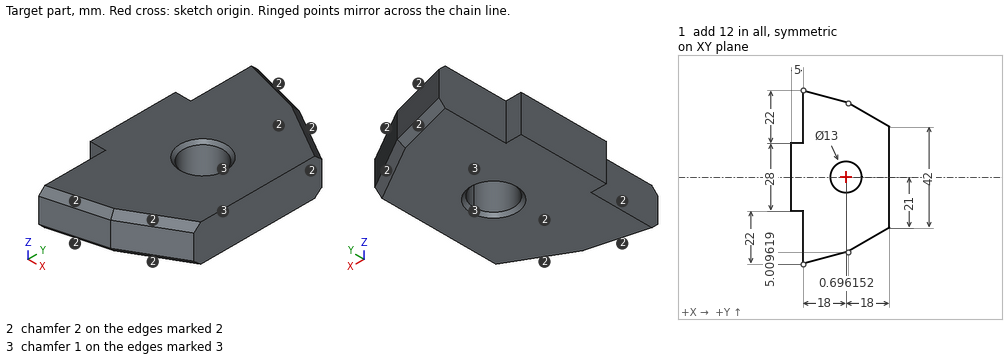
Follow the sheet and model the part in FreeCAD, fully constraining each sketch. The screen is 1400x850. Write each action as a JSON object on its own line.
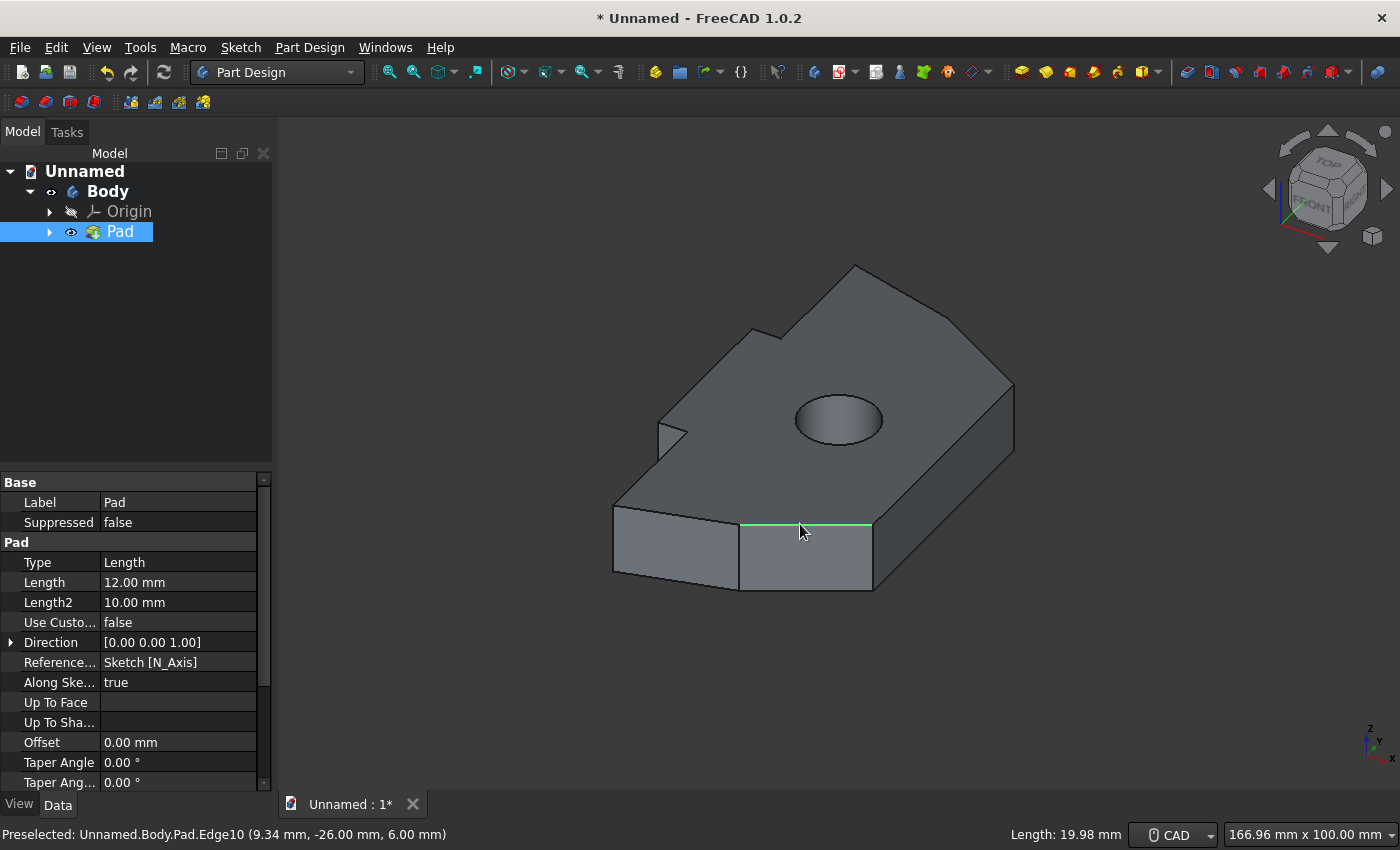
{"action": "left_click", "coordinate": [676, 514], "text": "ctrl"}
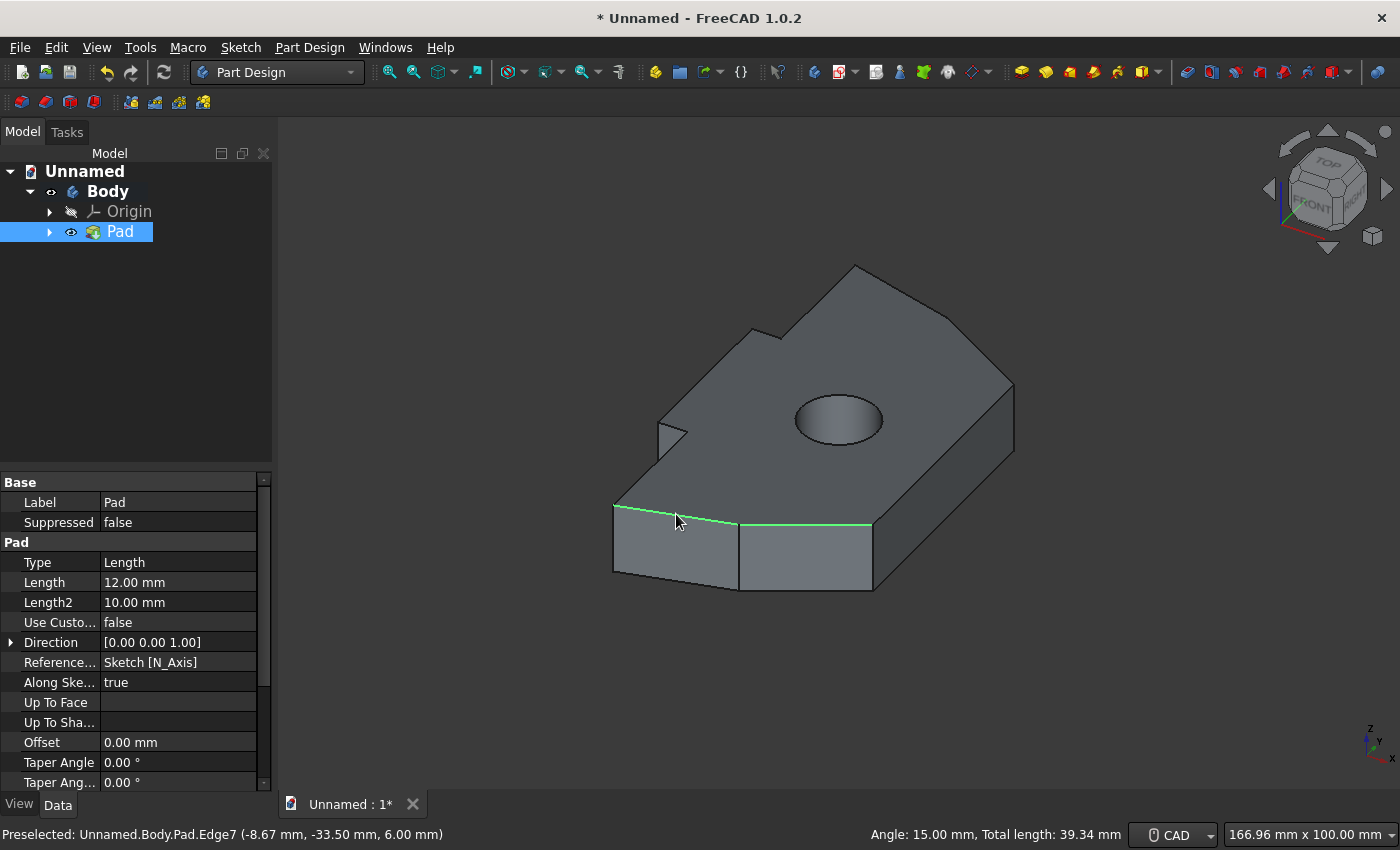
{"action": "key", "text": "0"}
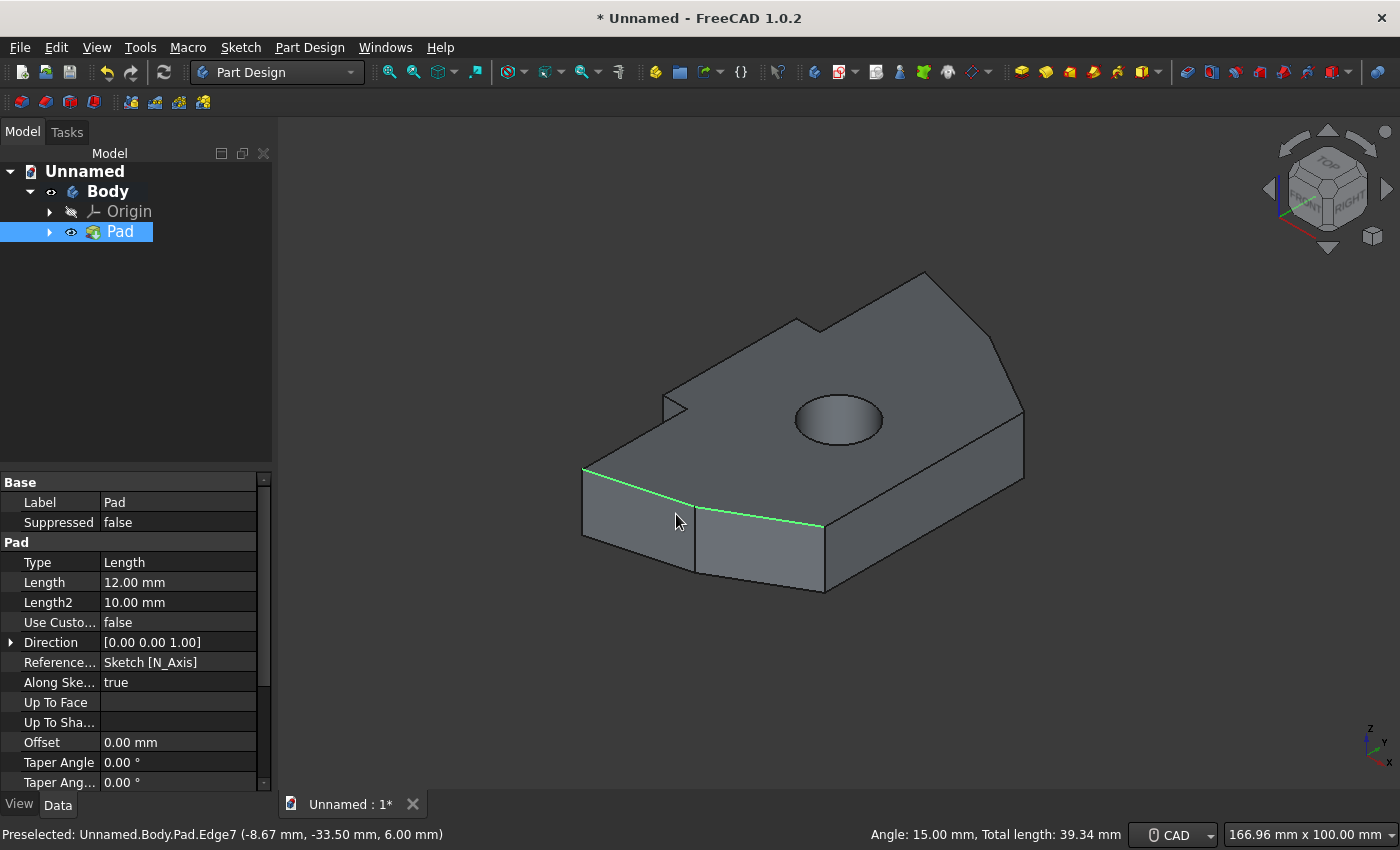
{"action": "key", "text": "2"}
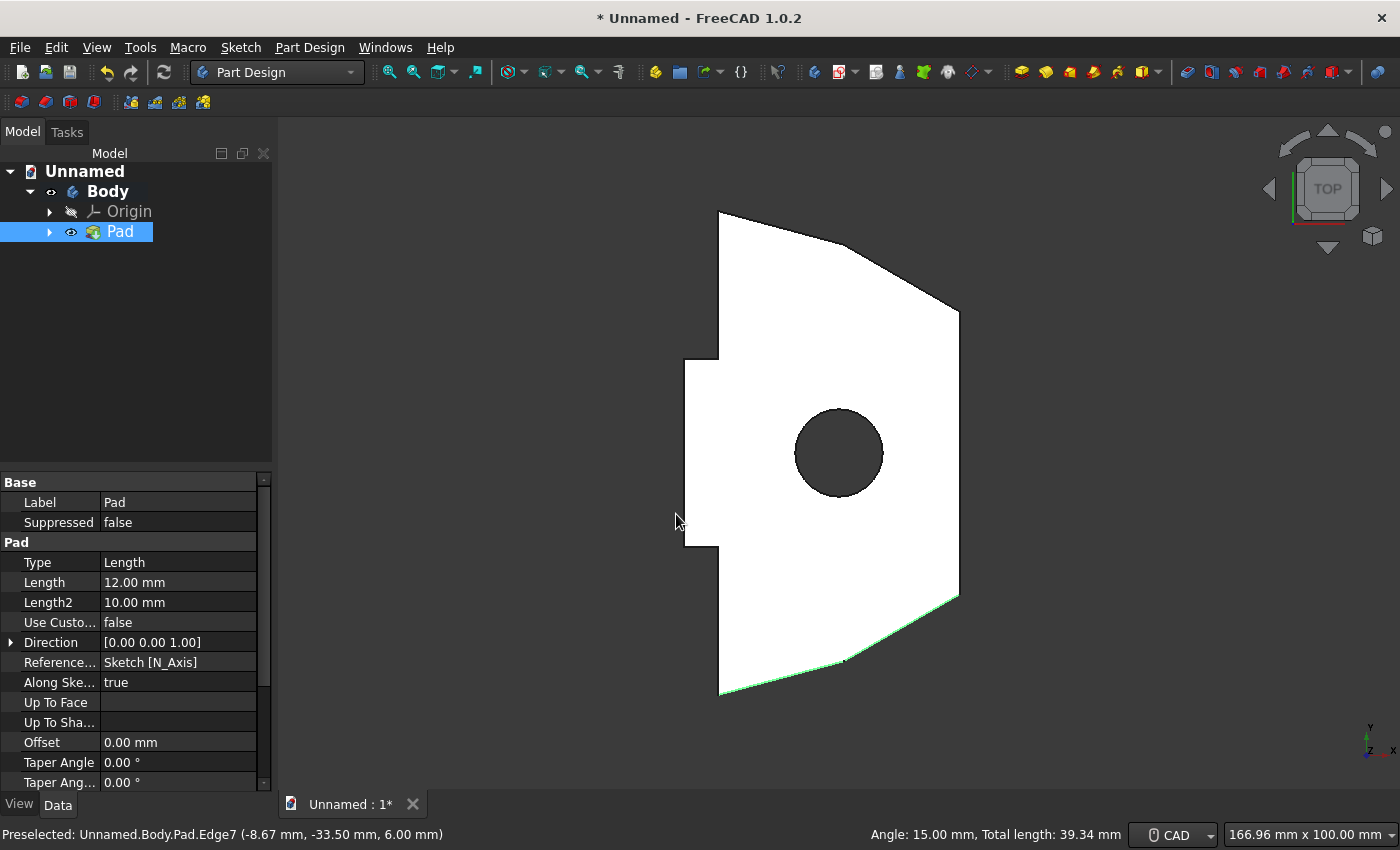
{"action": "left_click", "coordinate": [902, 277], "text": "ctrl"}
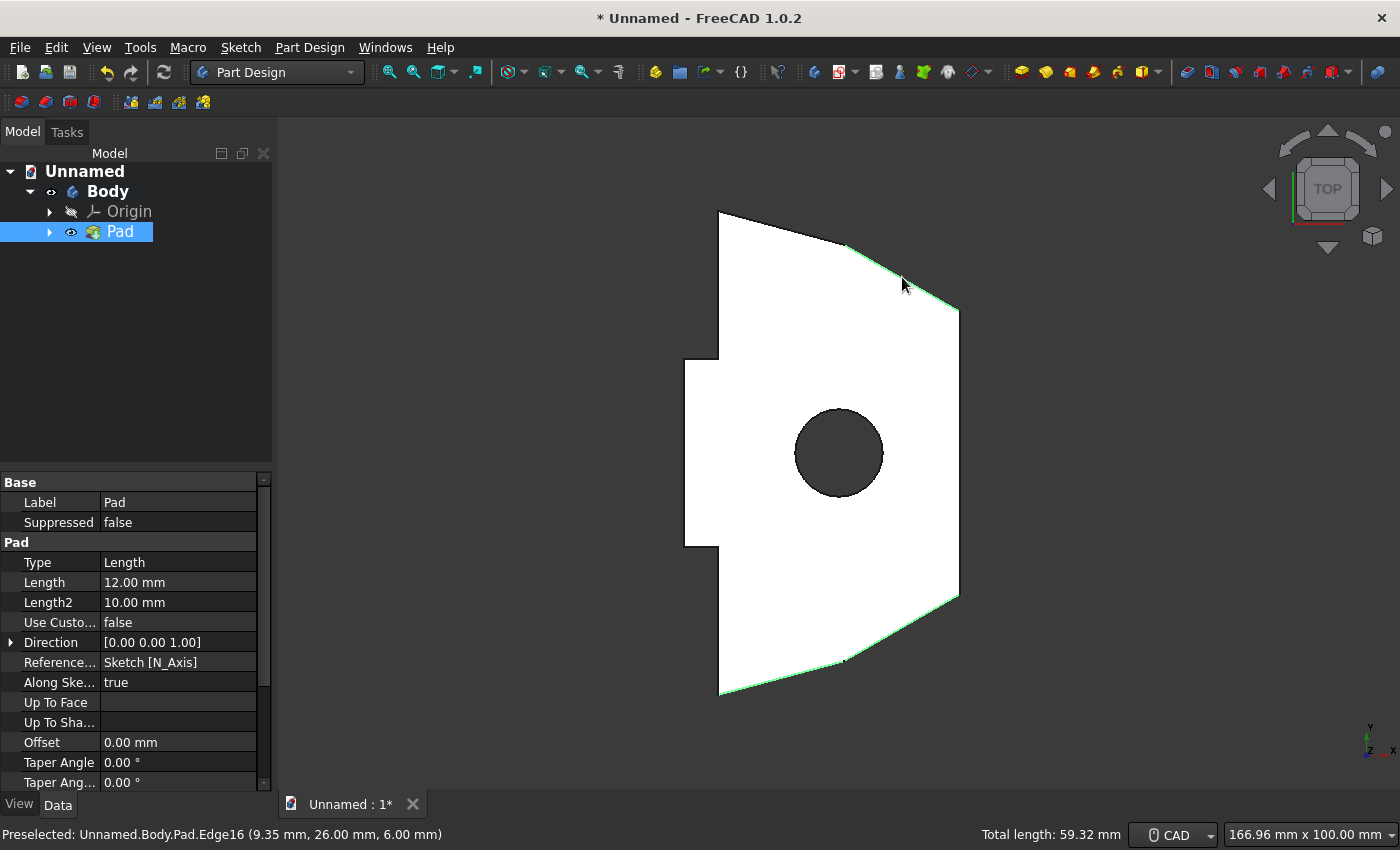
{"action": "left_click", "coordinate": [781, 227], "text": "ctrl"}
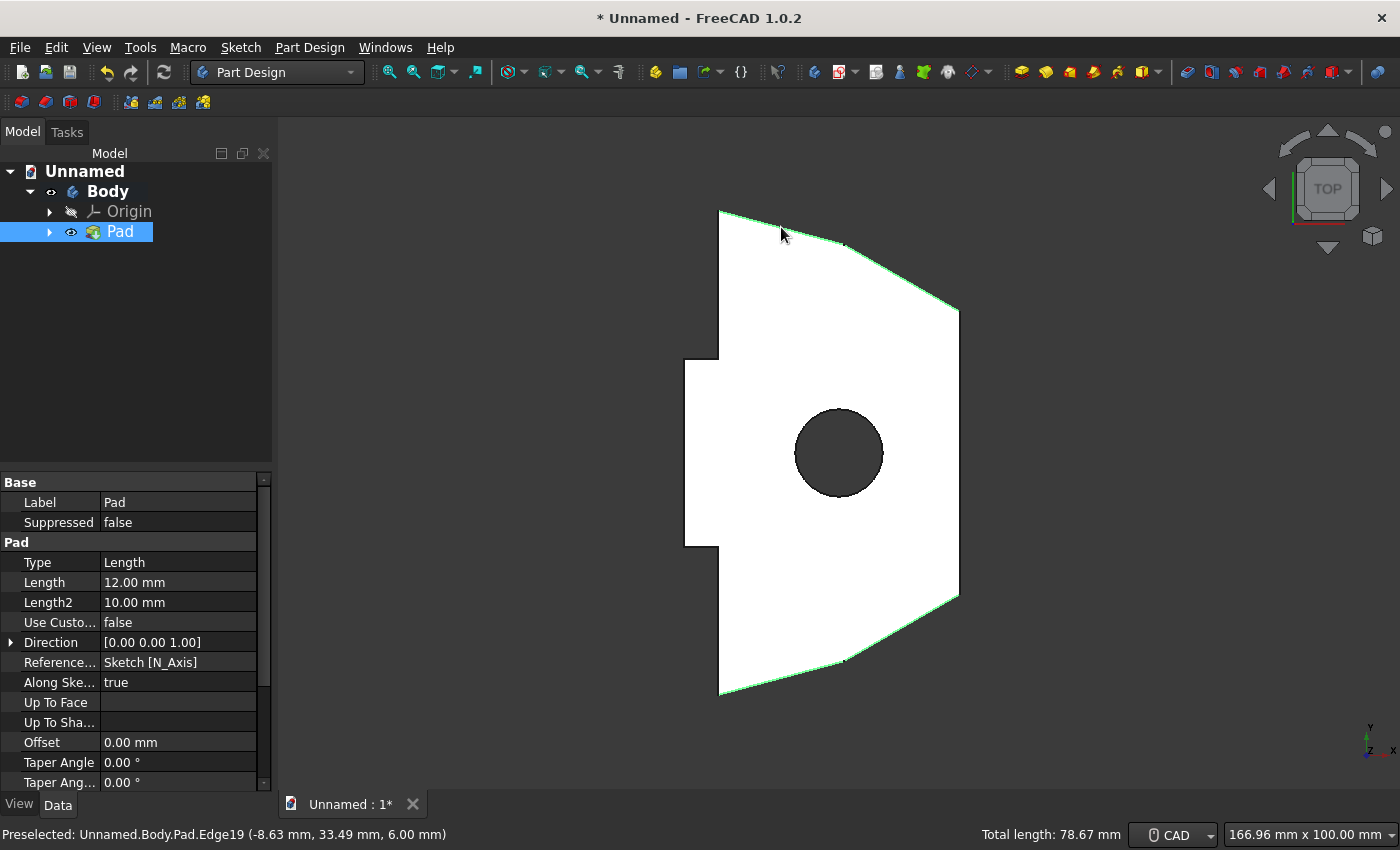
{"action": "key", "text": "1"}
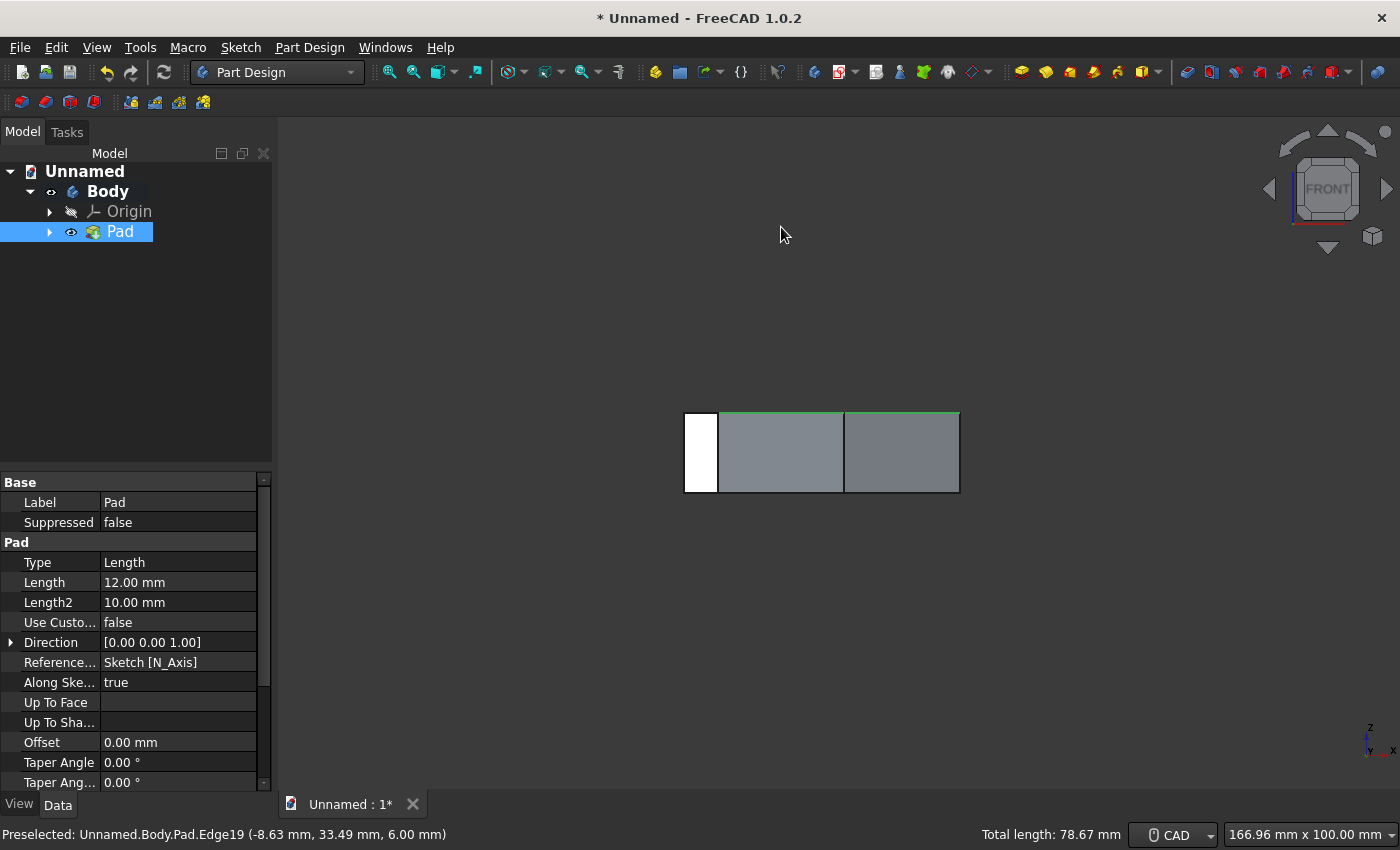
{"action": "key", "text": "v f"}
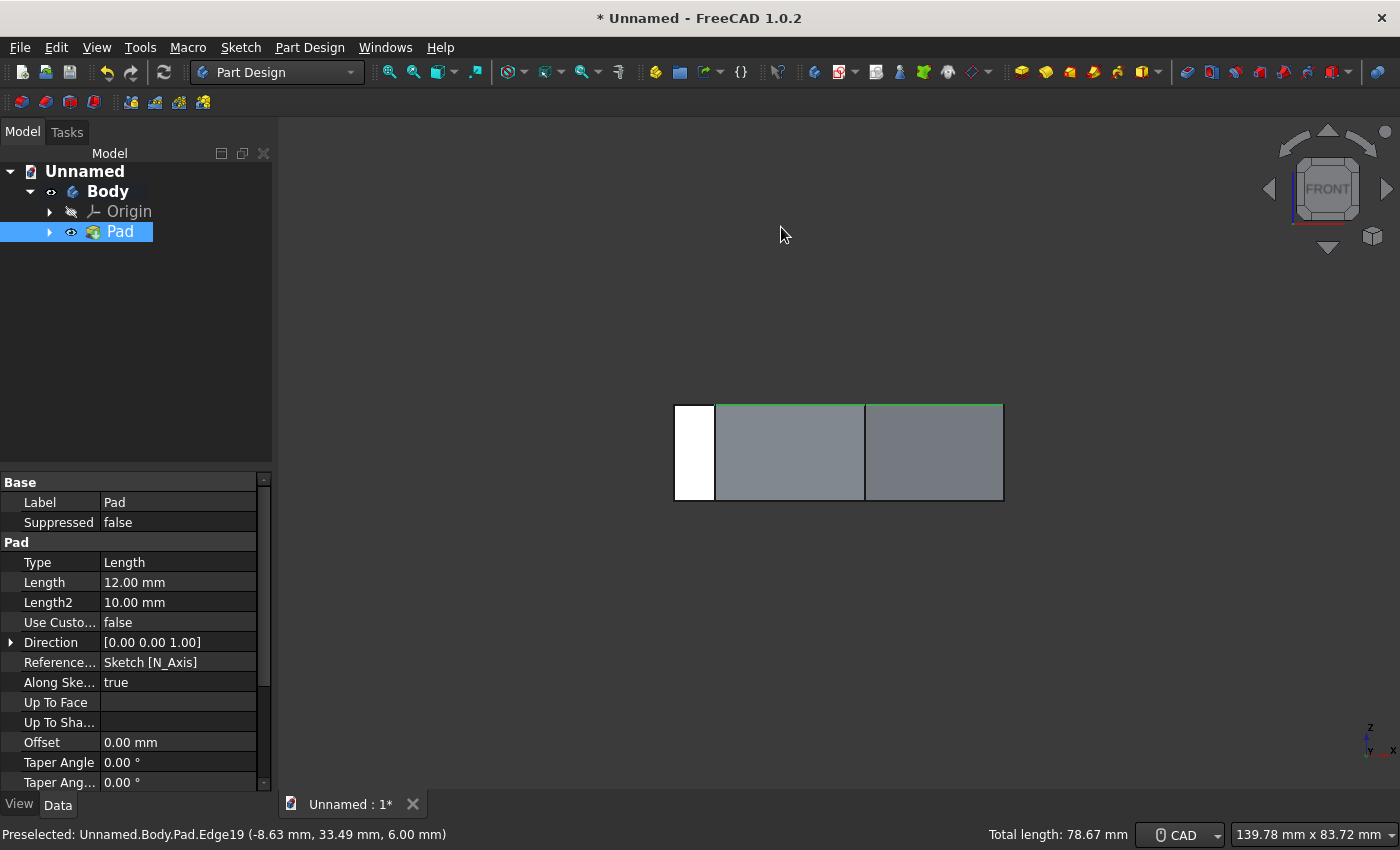
{"action": "left_click", "coordinate": [790, 500], "text": "ctrl"}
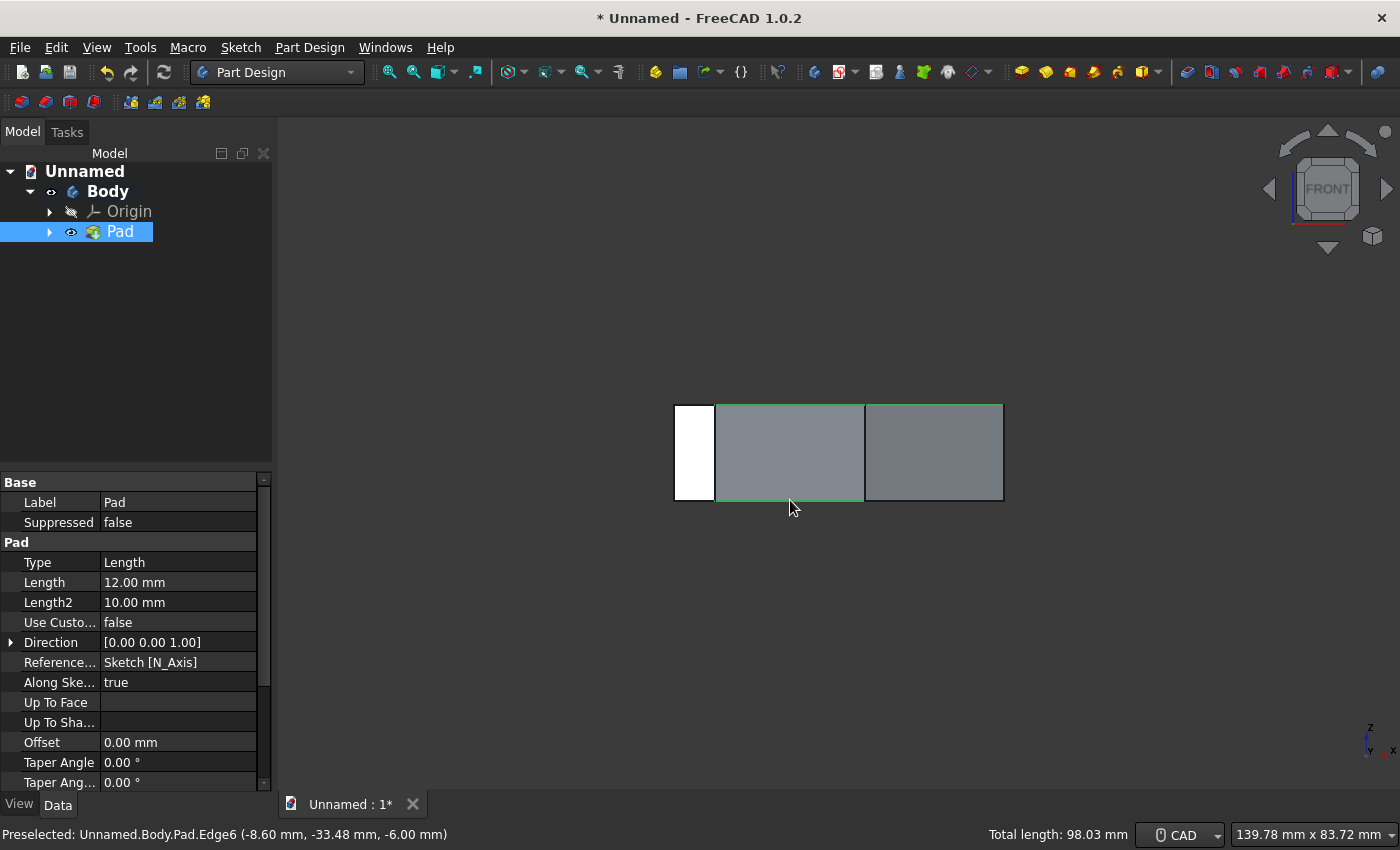
{"action": "left_click", "coordinate": [934, 500], "text": "ctrl"}